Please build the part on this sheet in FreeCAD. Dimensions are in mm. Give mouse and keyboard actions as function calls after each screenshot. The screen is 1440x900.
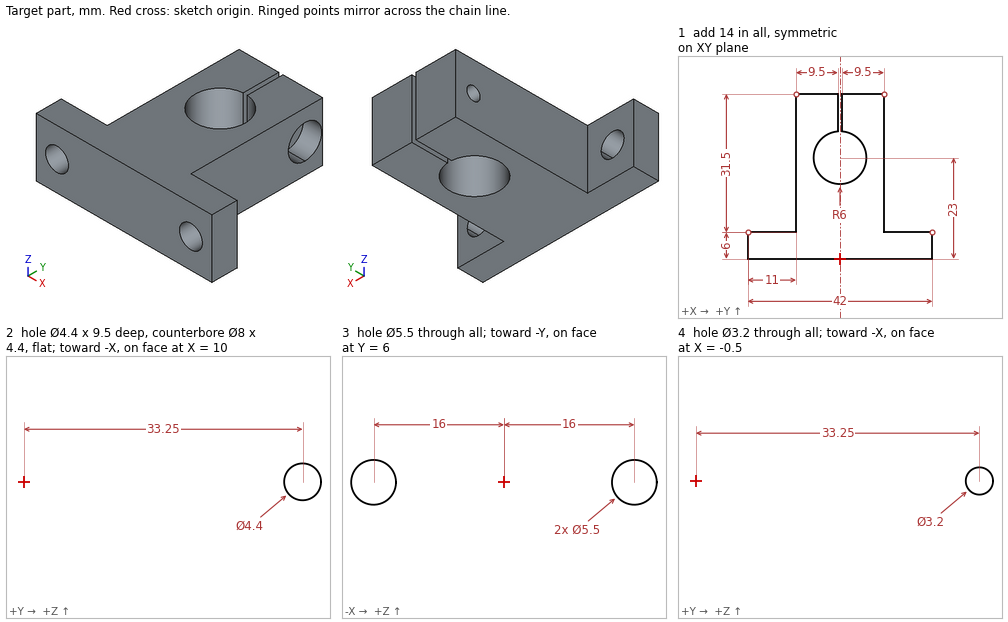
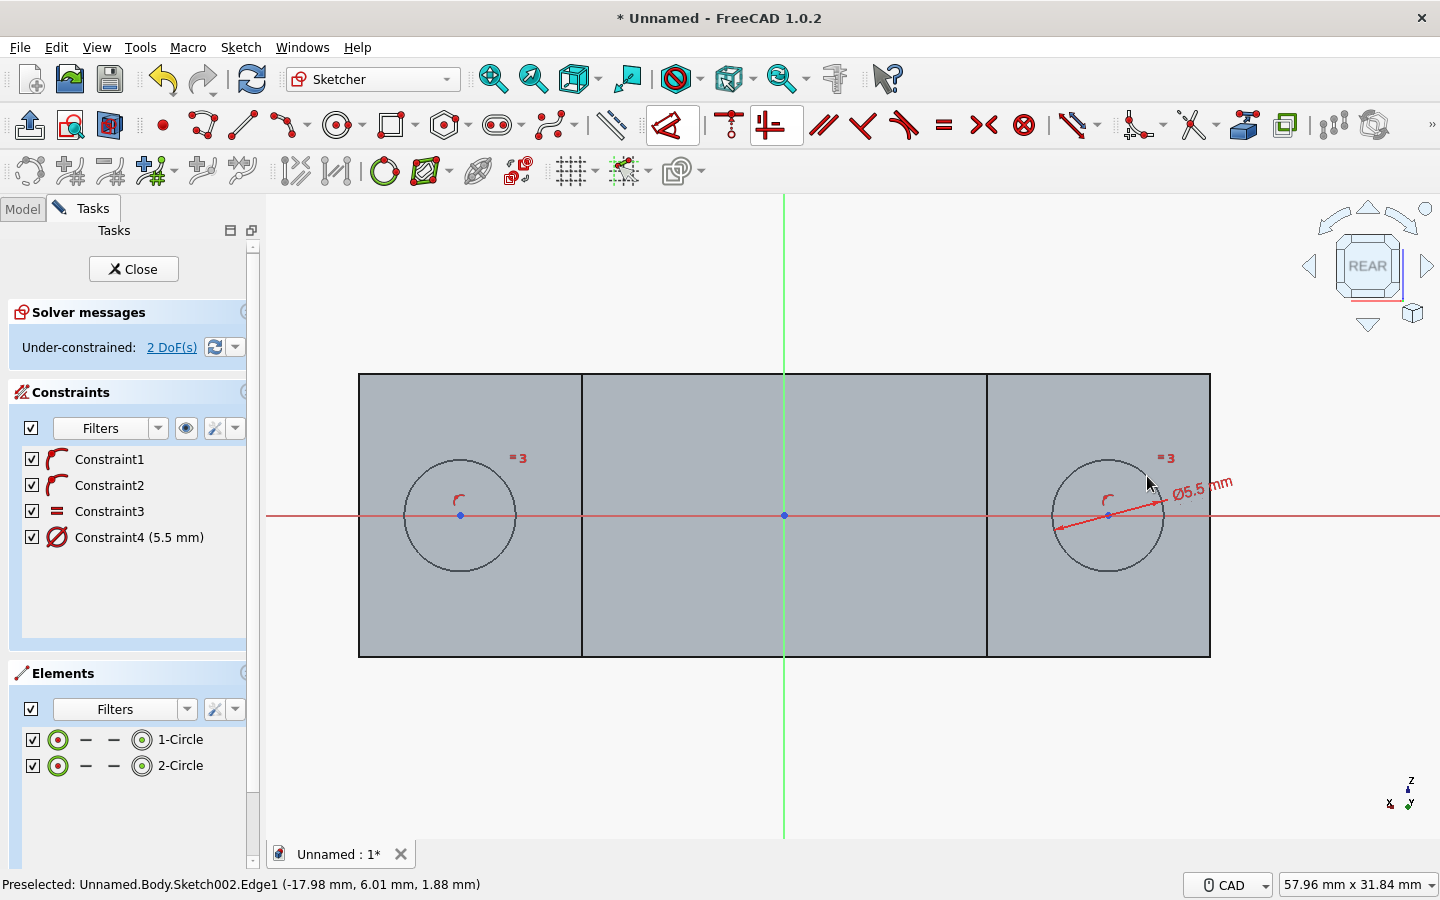
click(1108, 516)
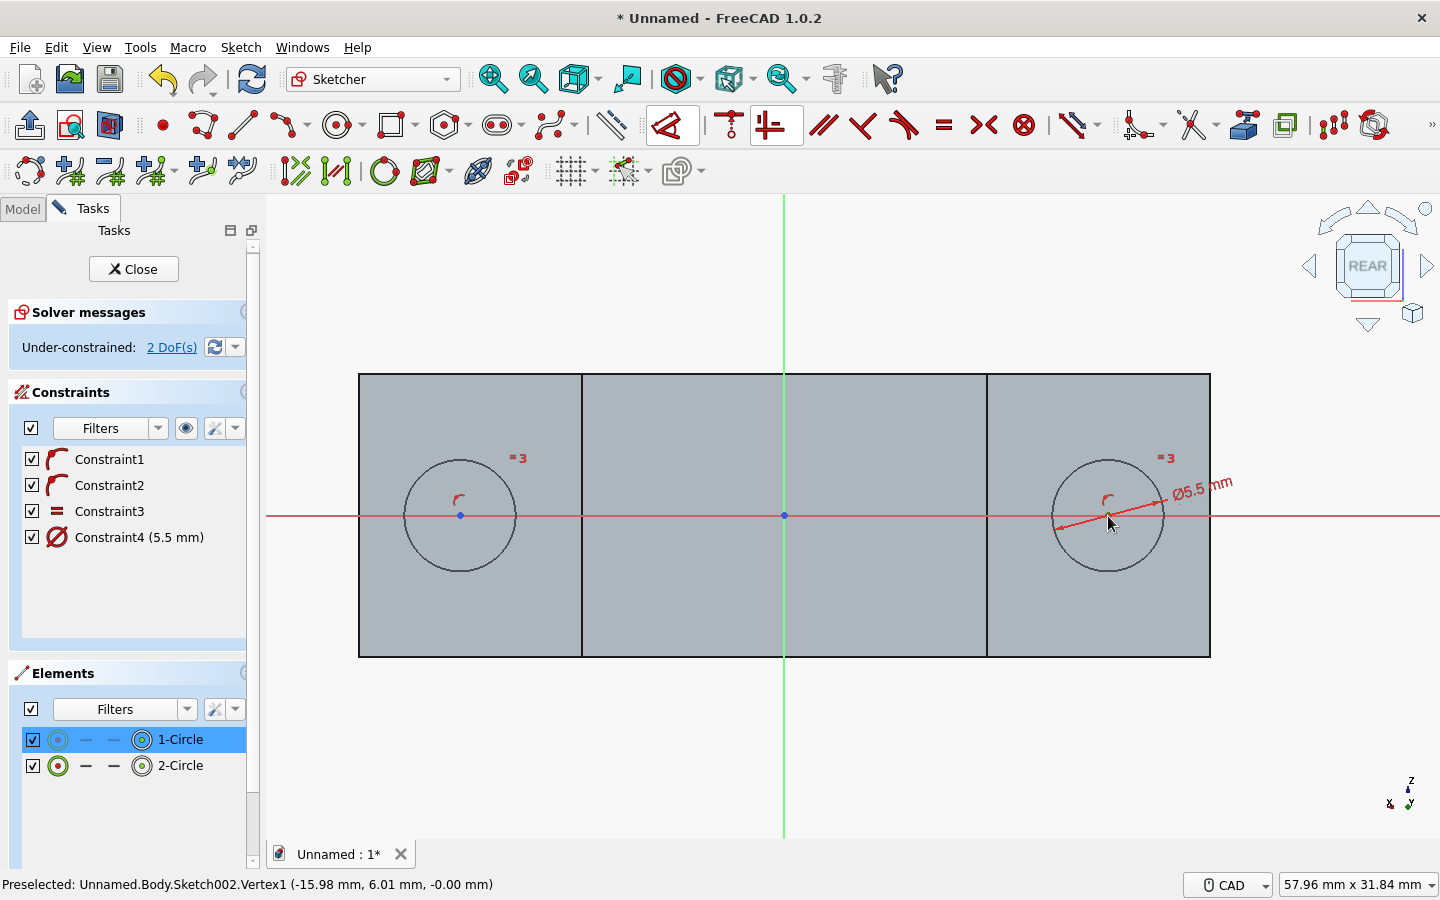
key(l)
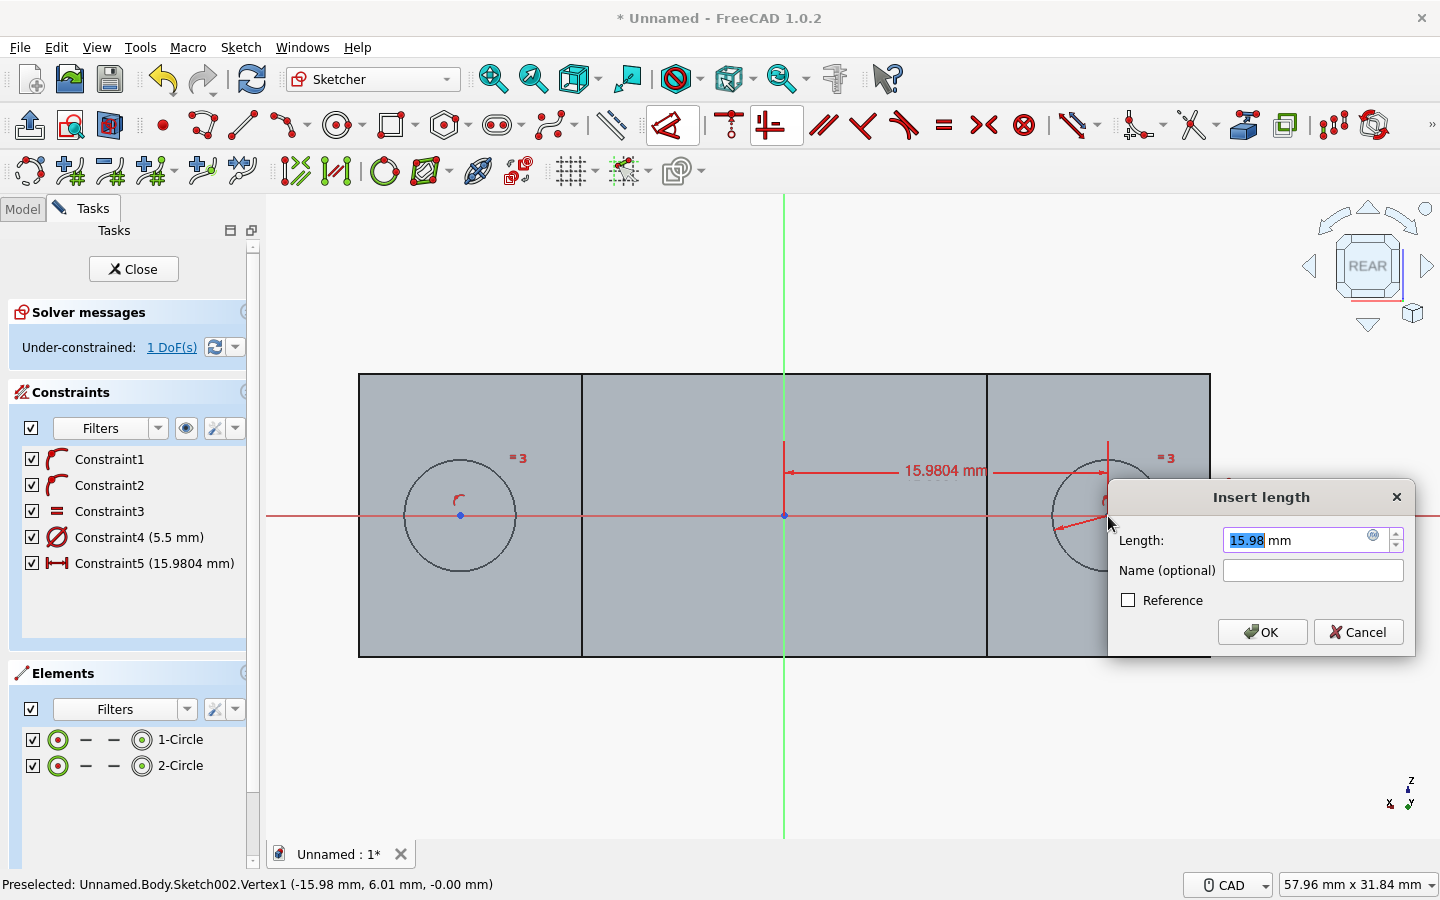
text(16)
key(Return)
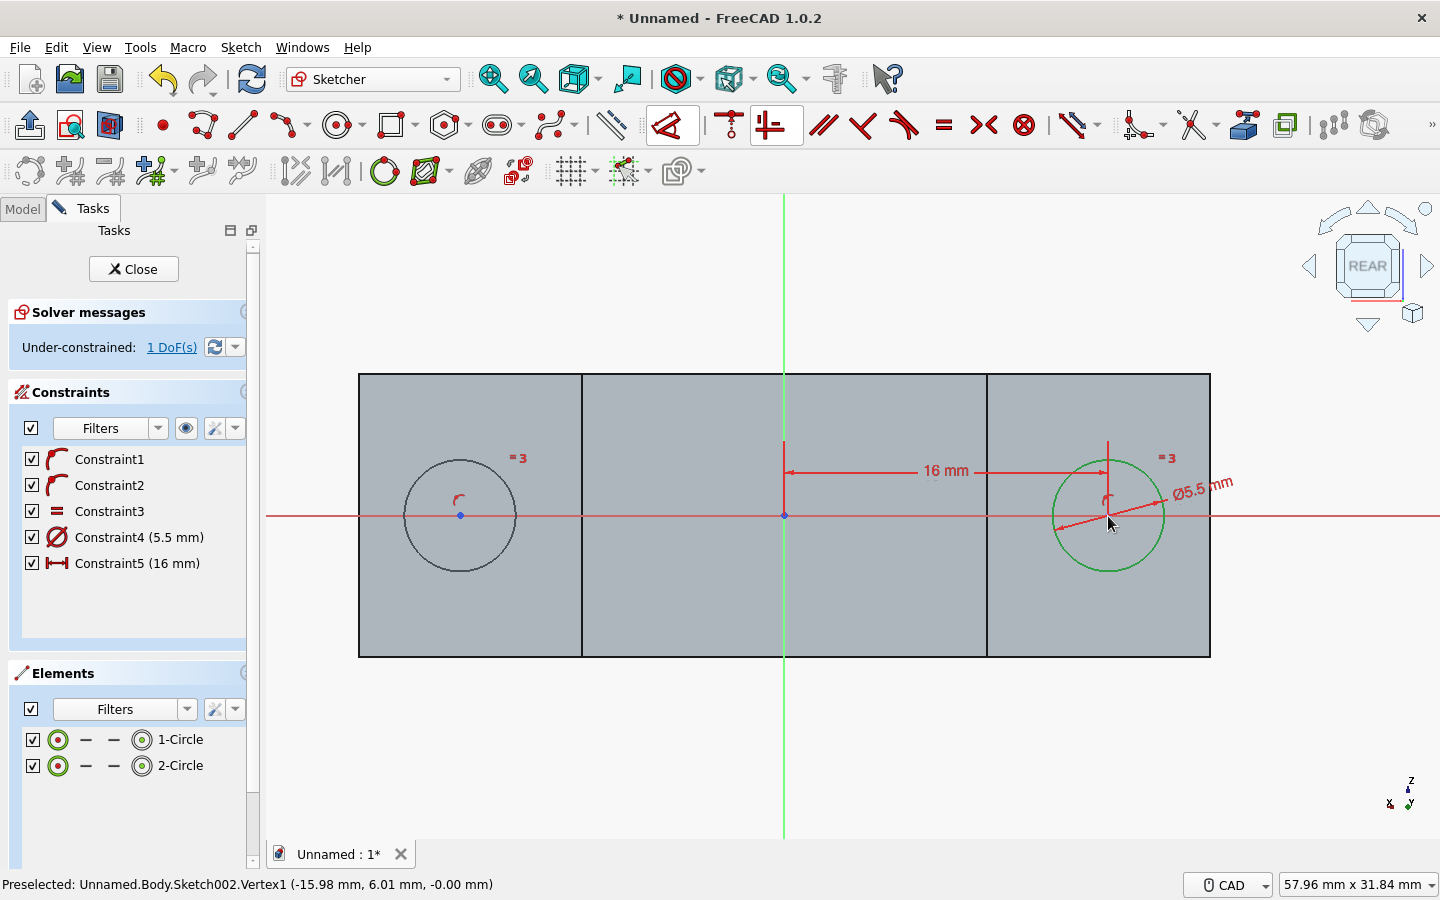
click(460, 516)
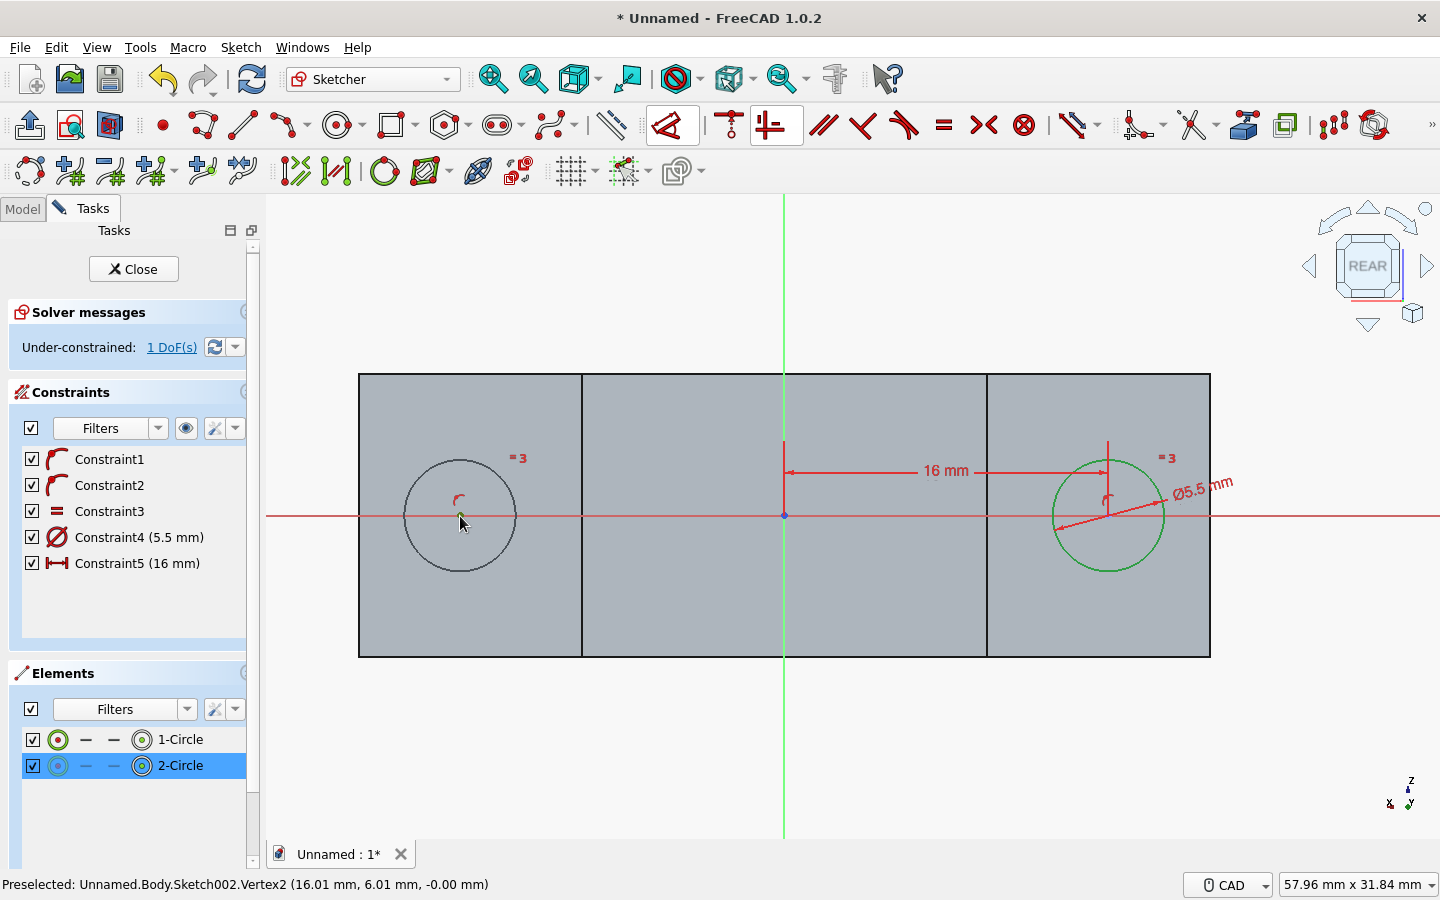
click(694, 126)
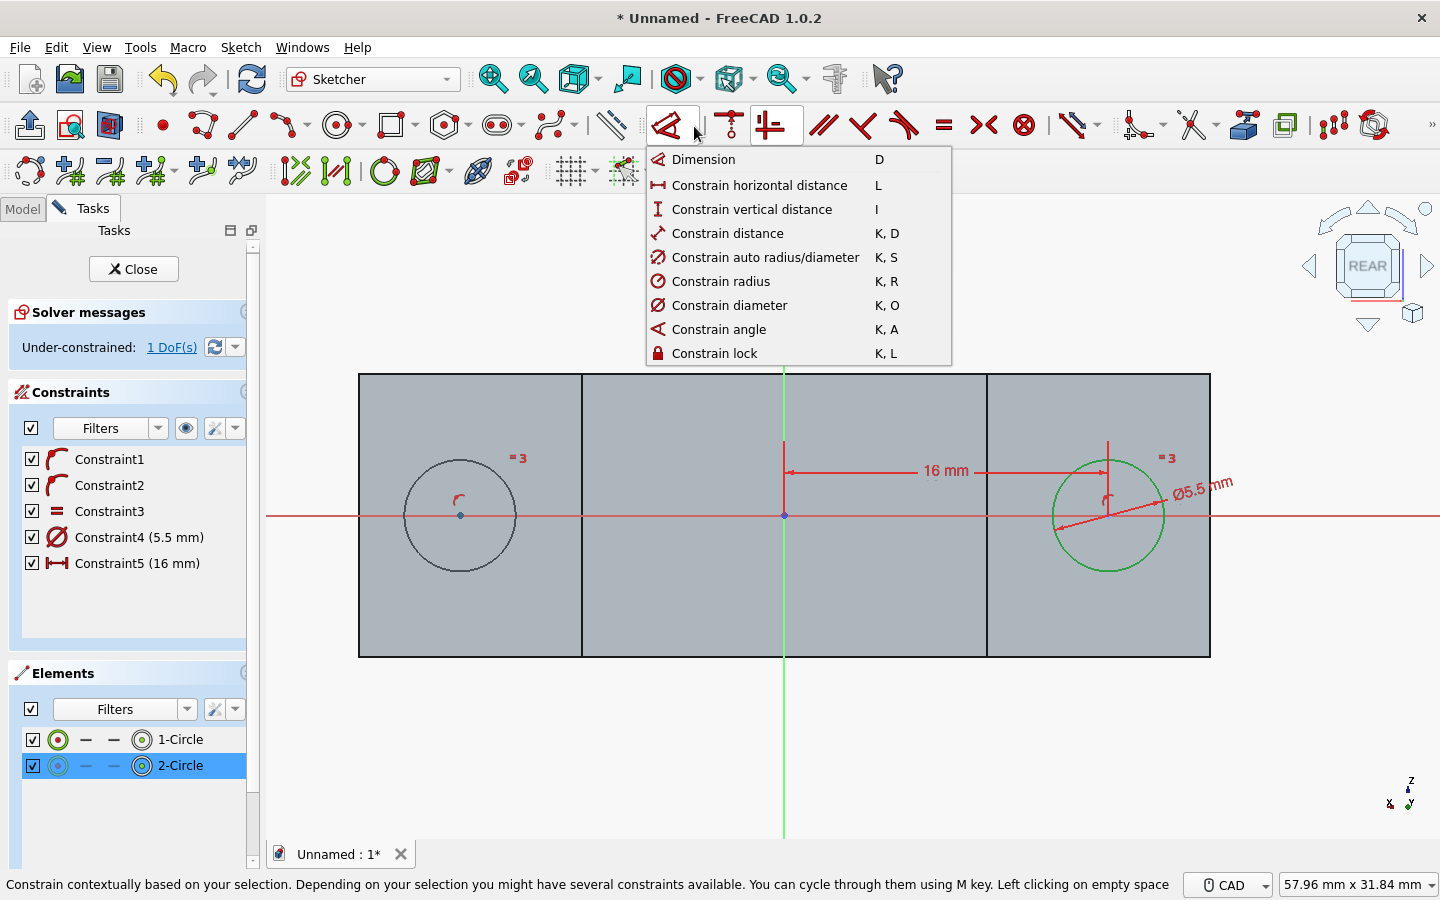
click(799, 185)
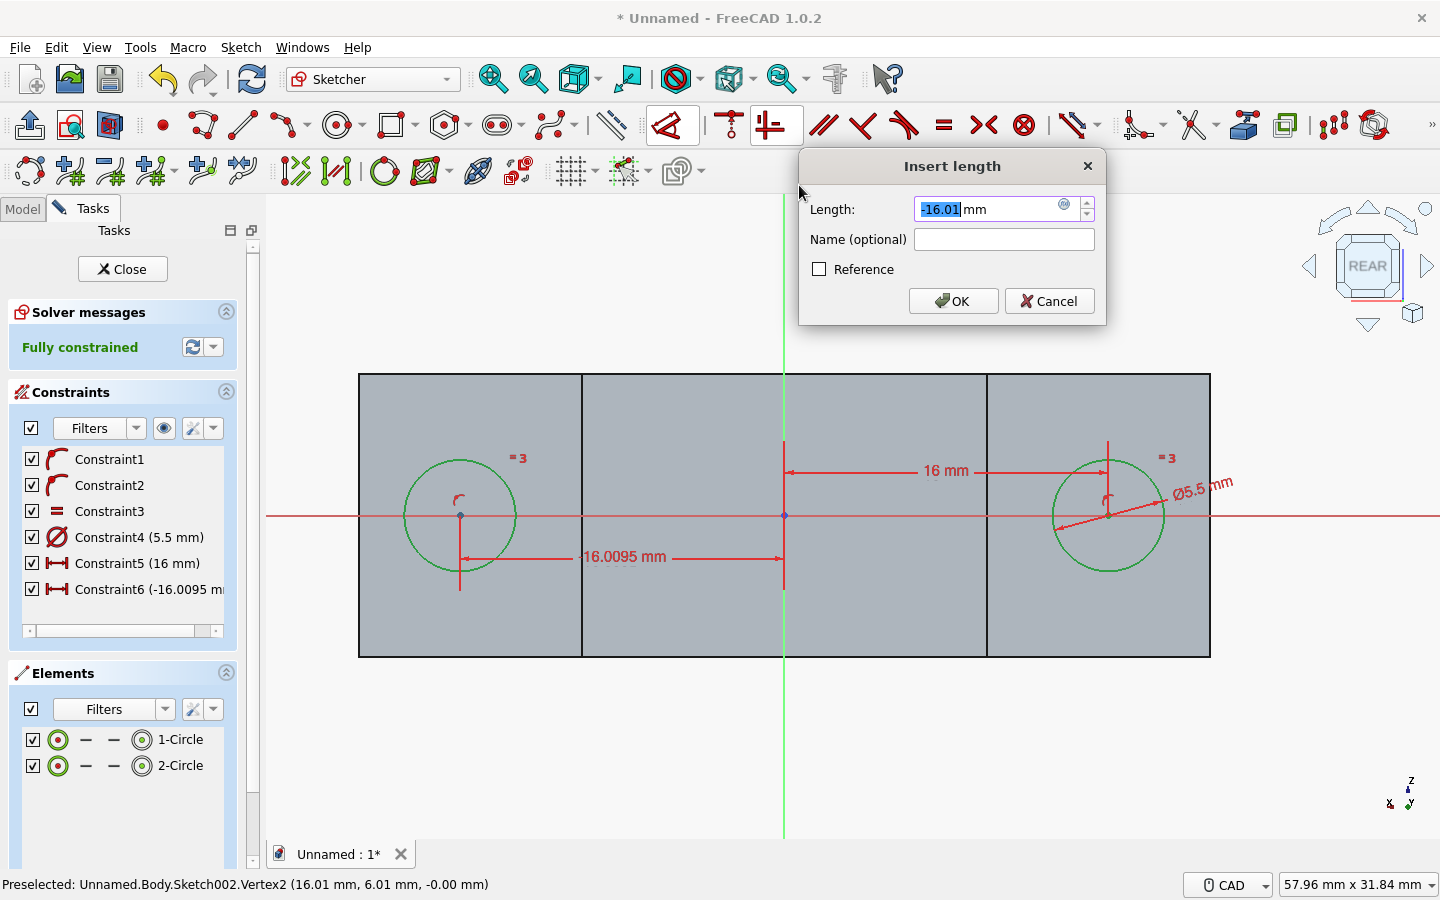
text(-16)
key(Return)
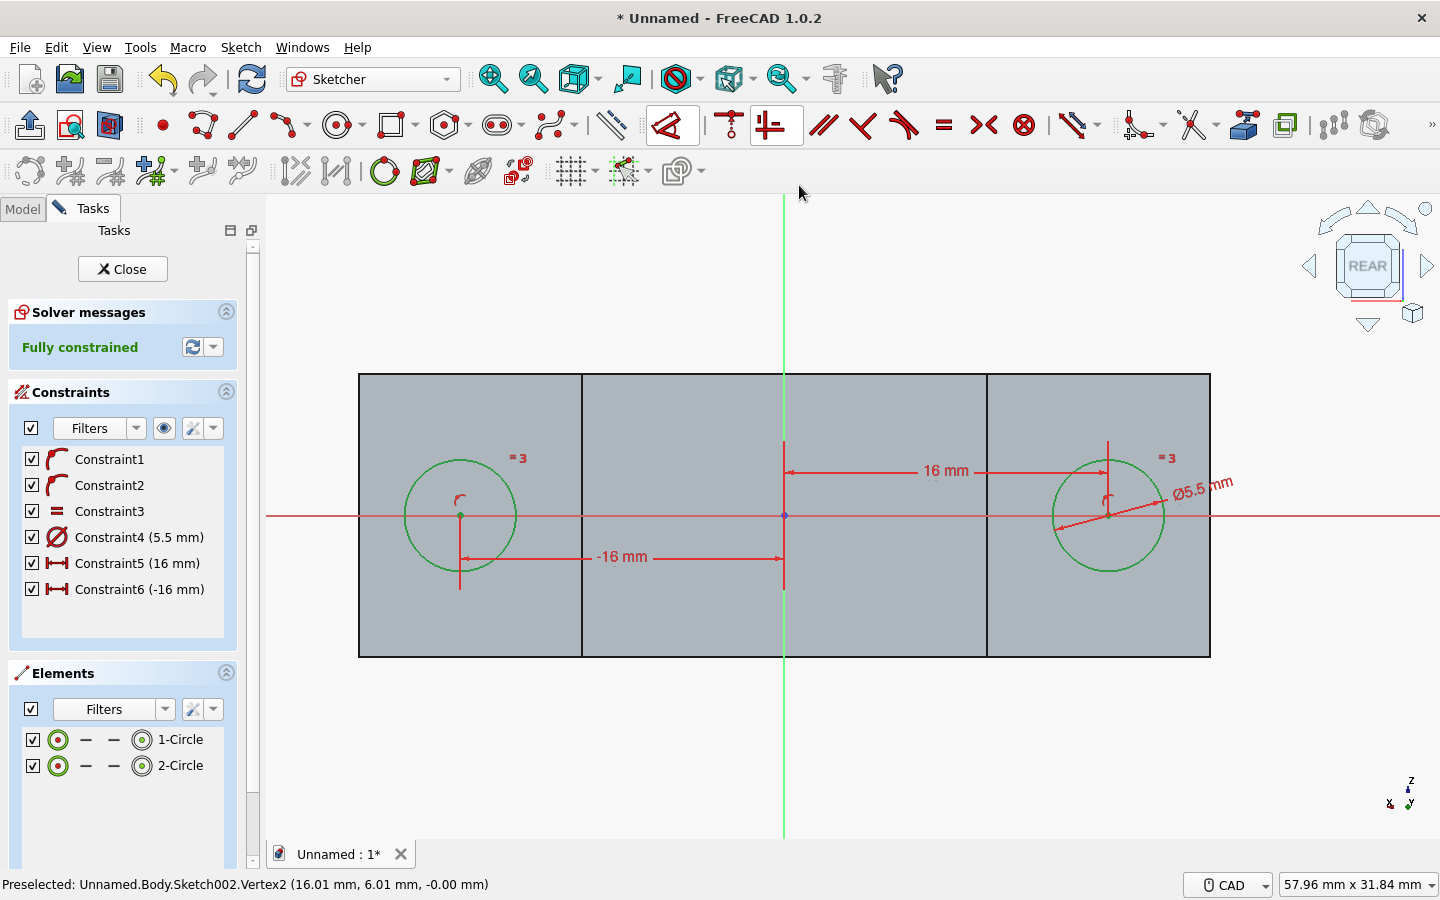
click(123, 269)